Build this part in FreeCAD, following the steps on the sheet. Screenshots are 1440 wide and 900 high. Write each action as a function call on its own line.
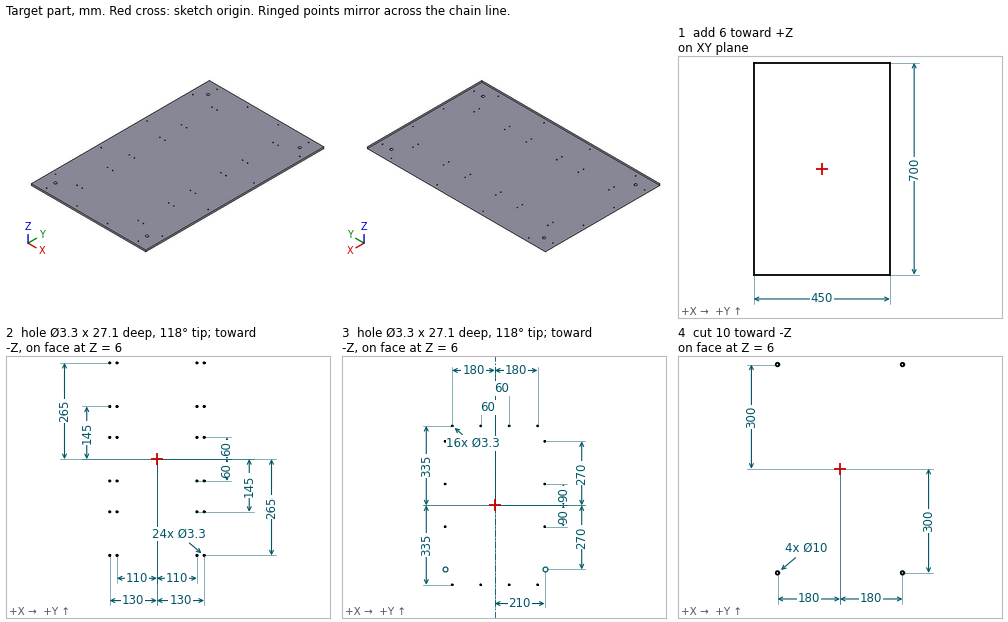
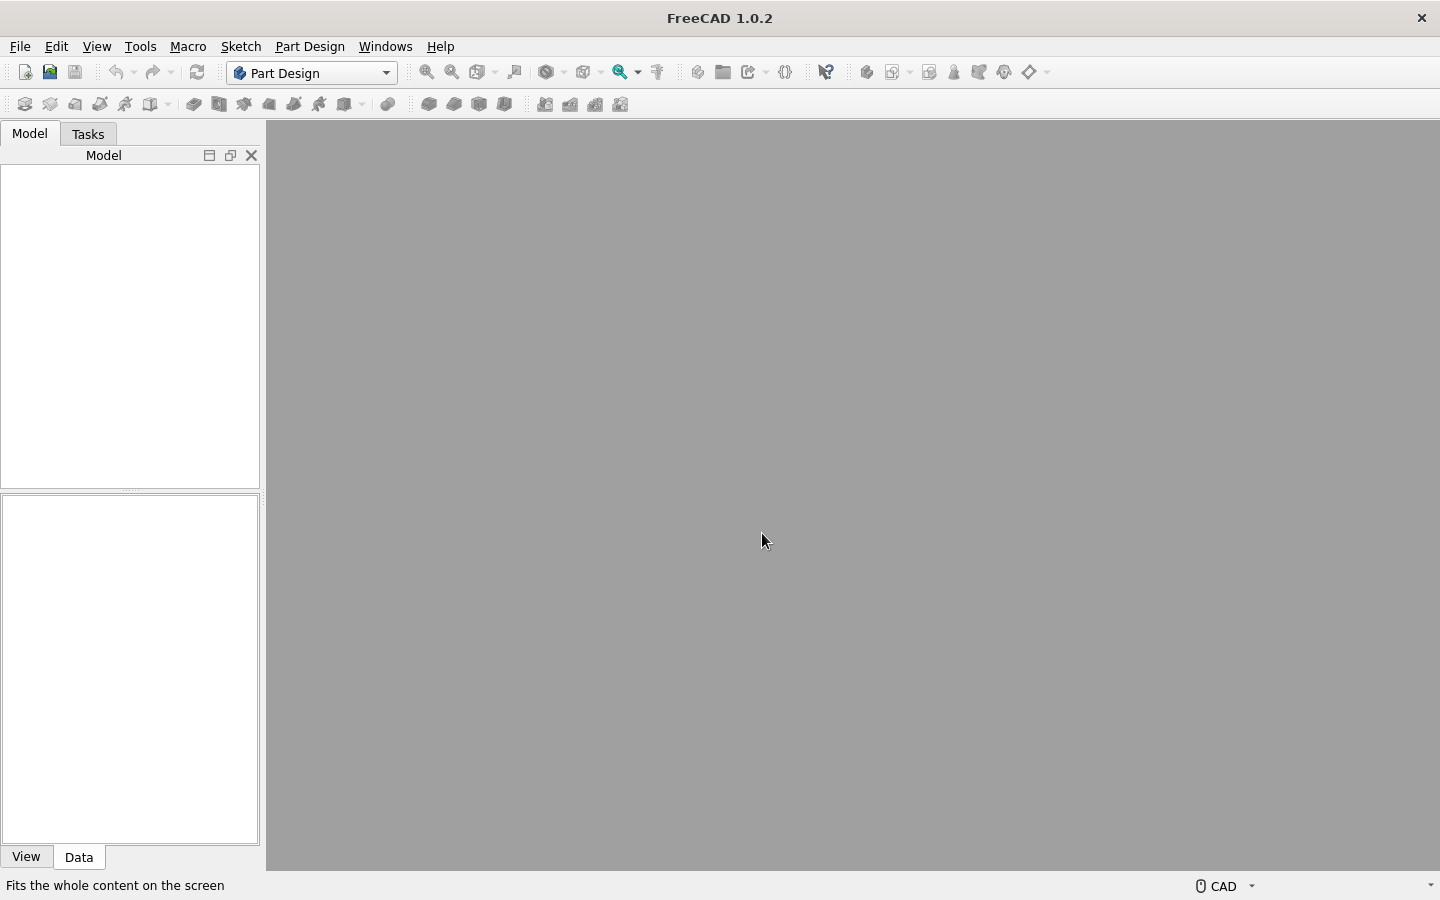
click(25, 72)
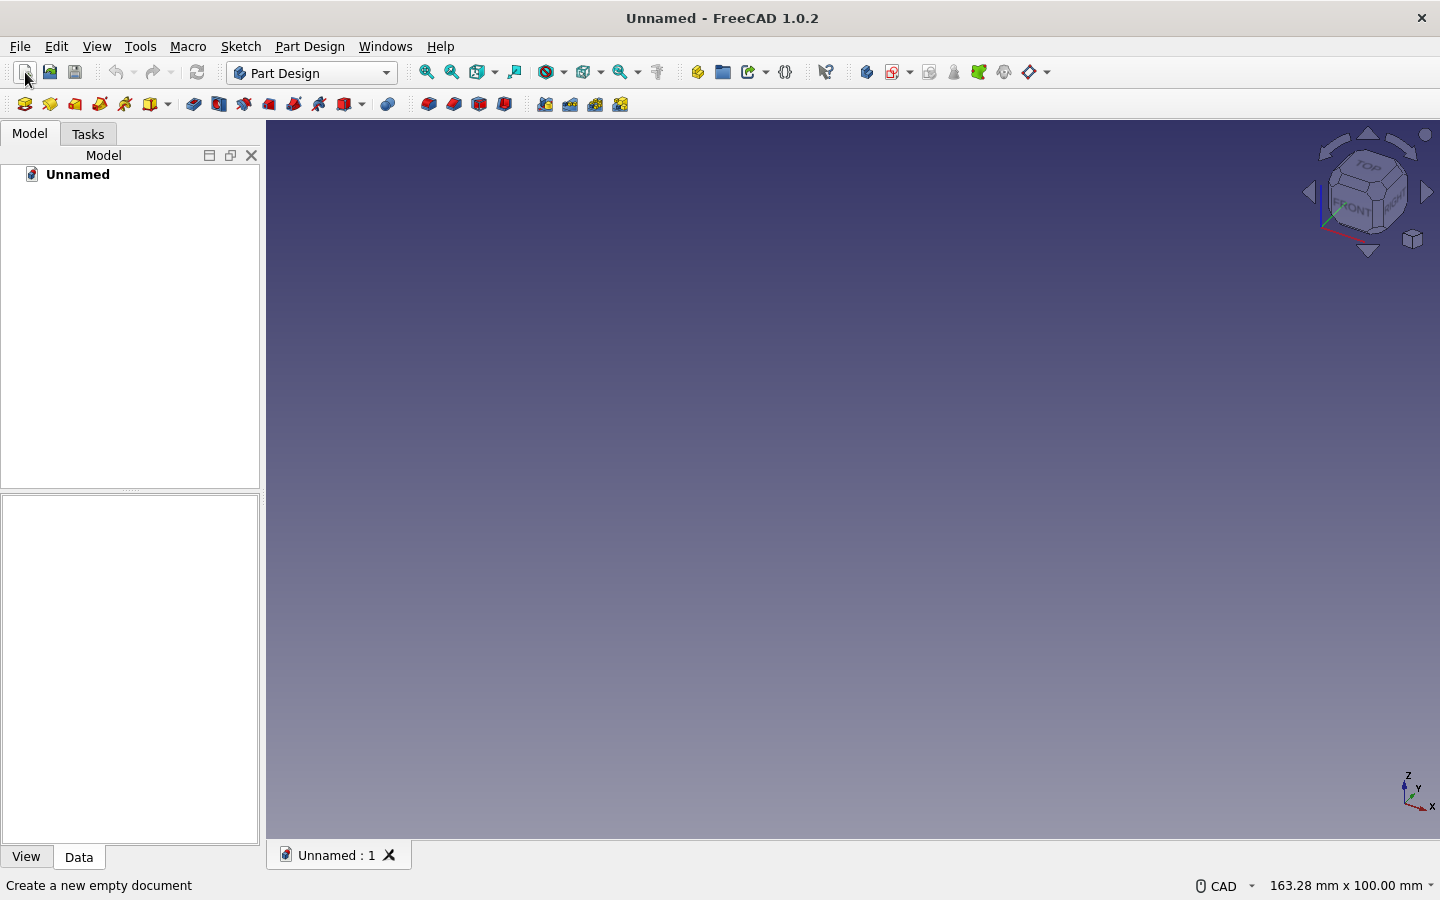
click(892, 72)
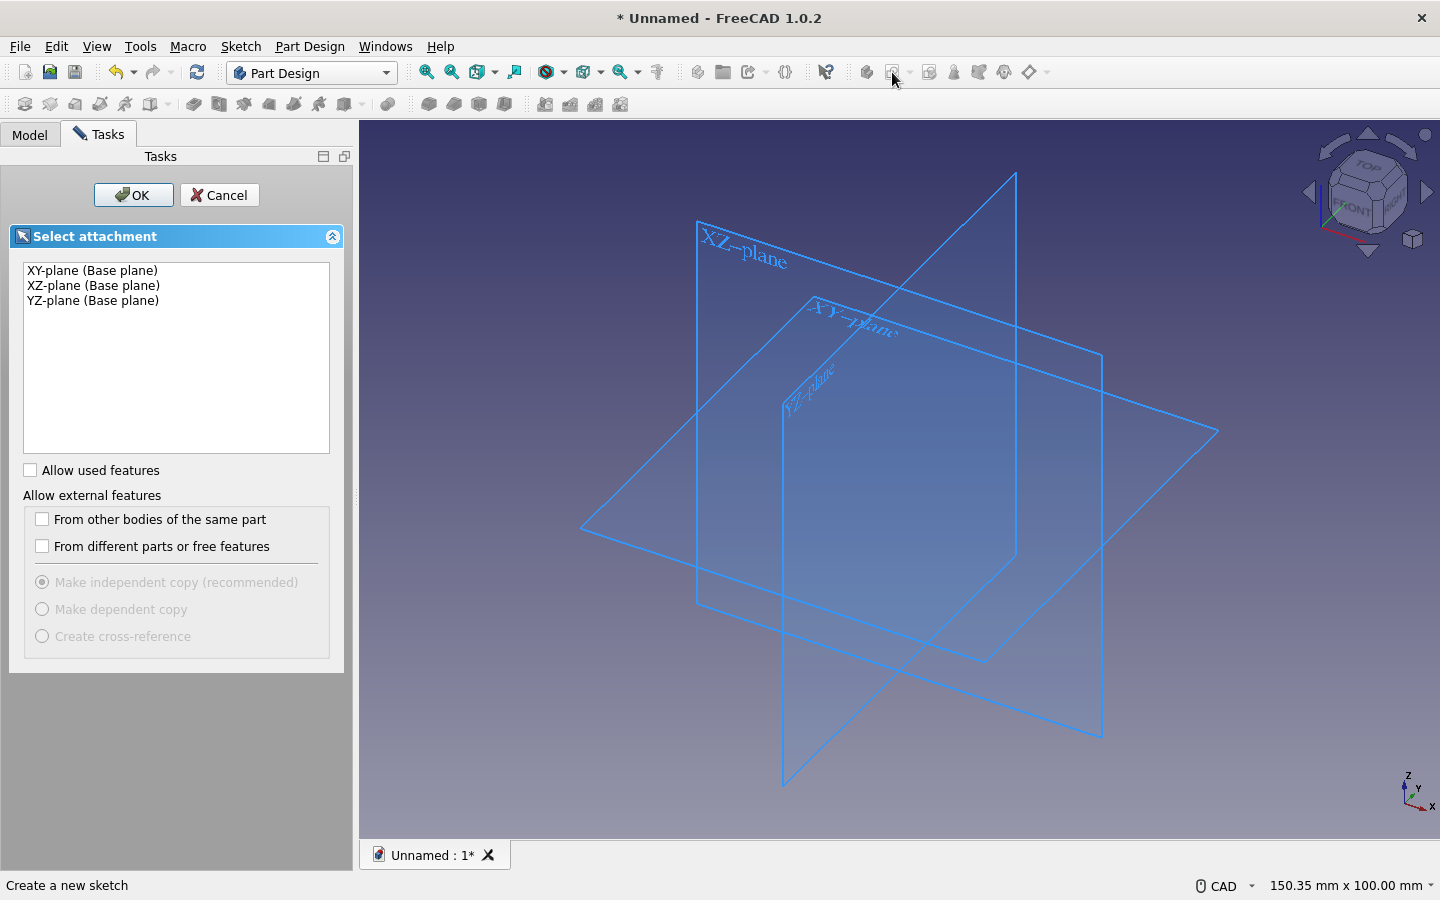
click(84, 270)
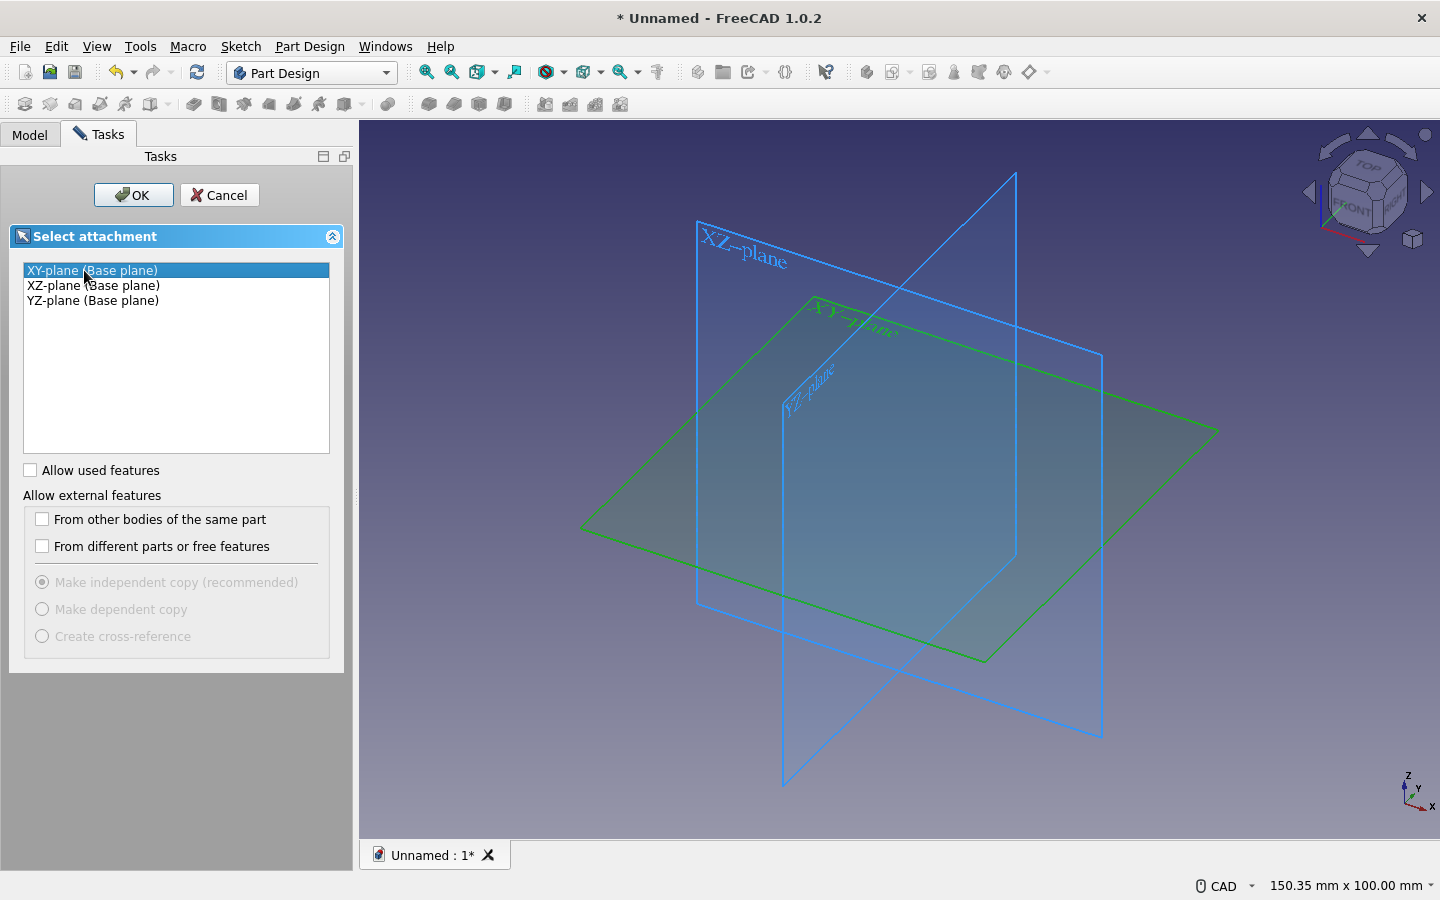
click(134, 195)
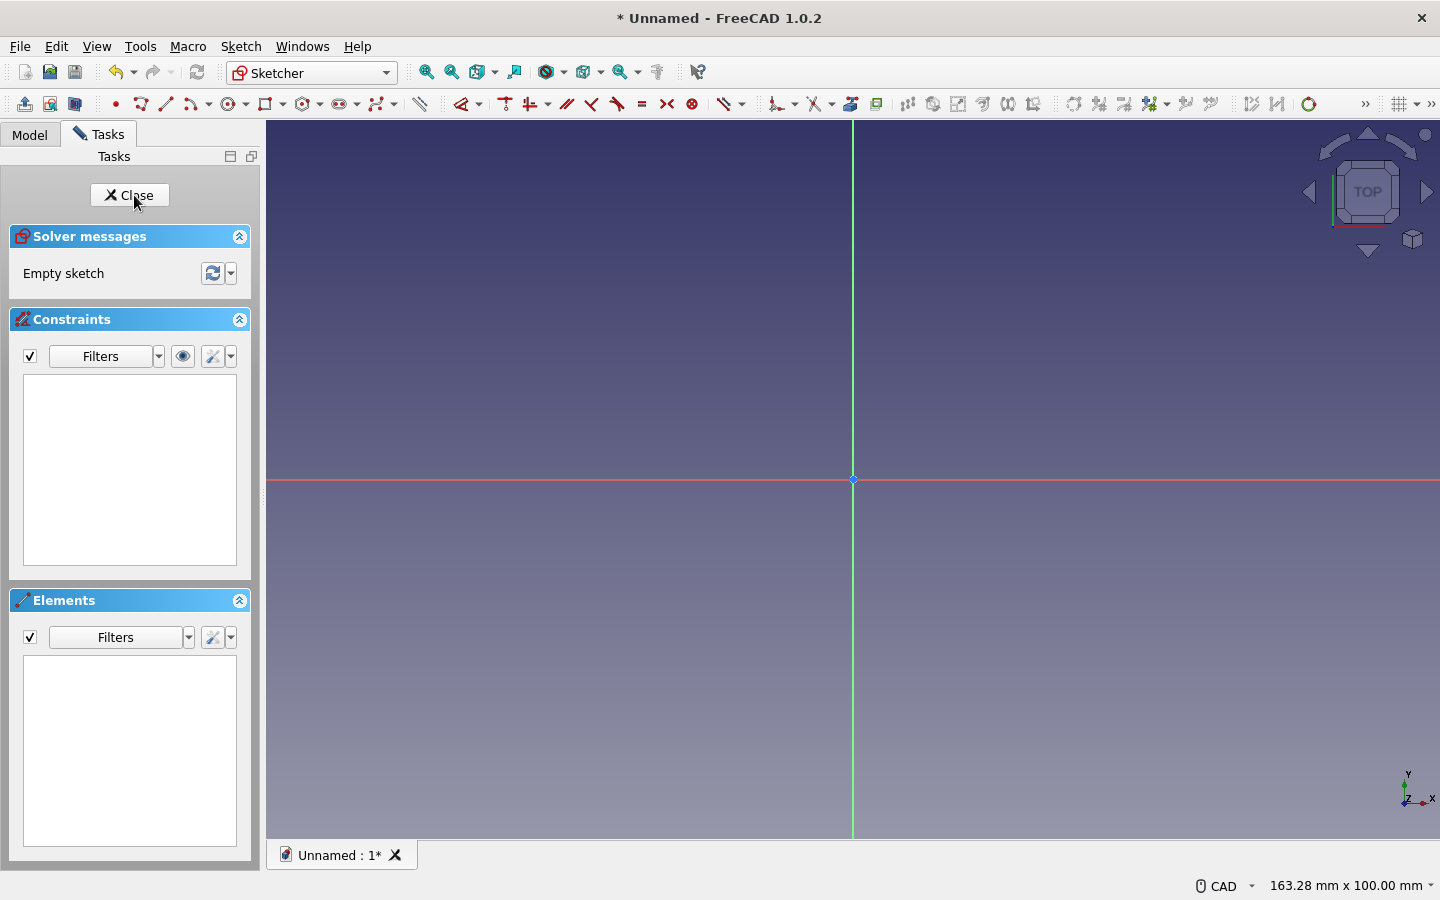
scroll(778, 479, down, 12)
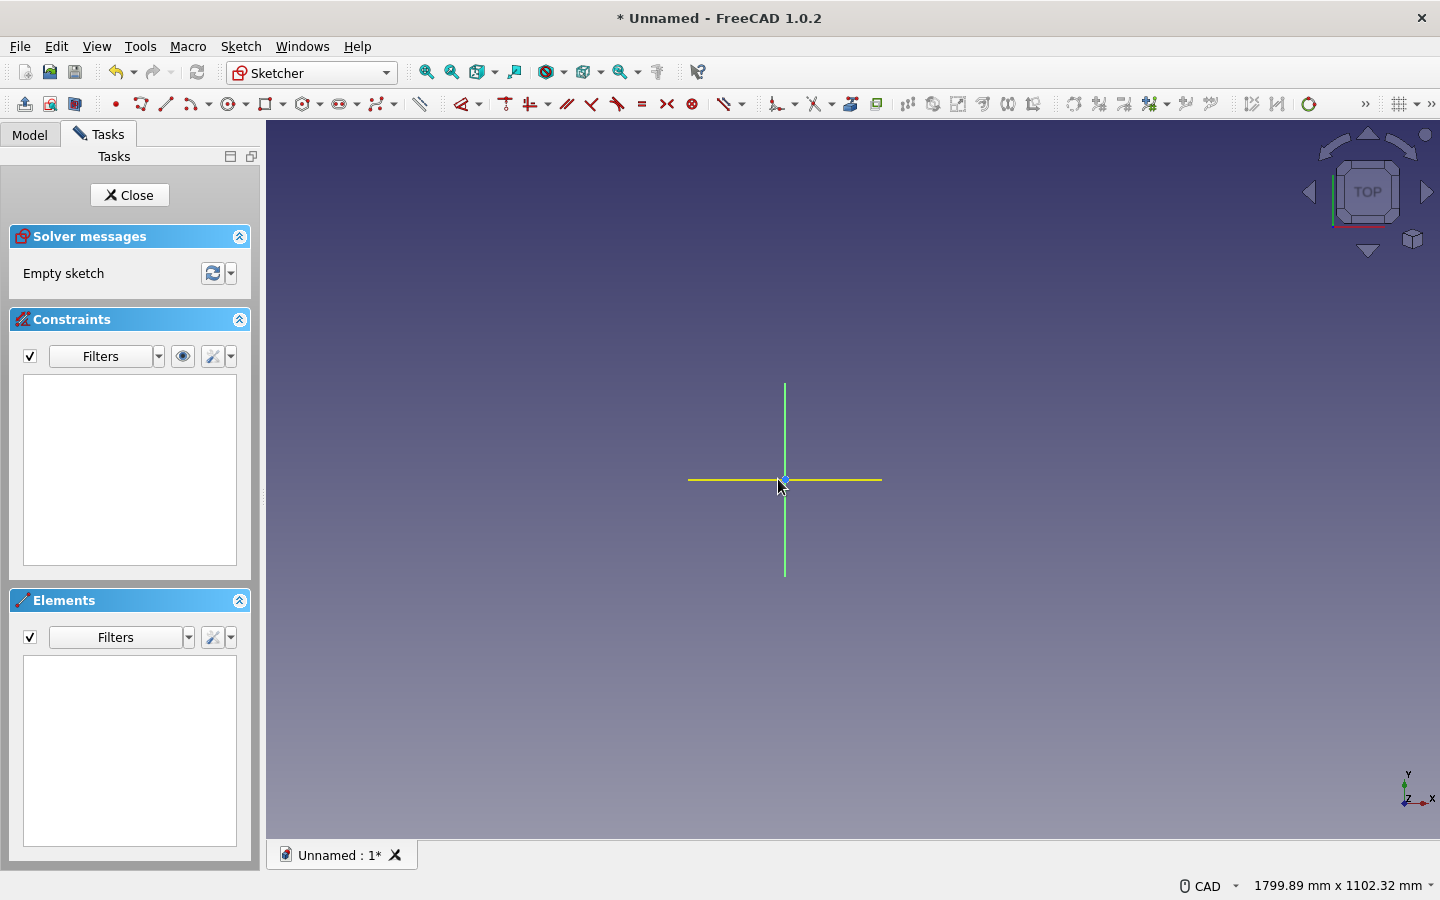
click(282, 104)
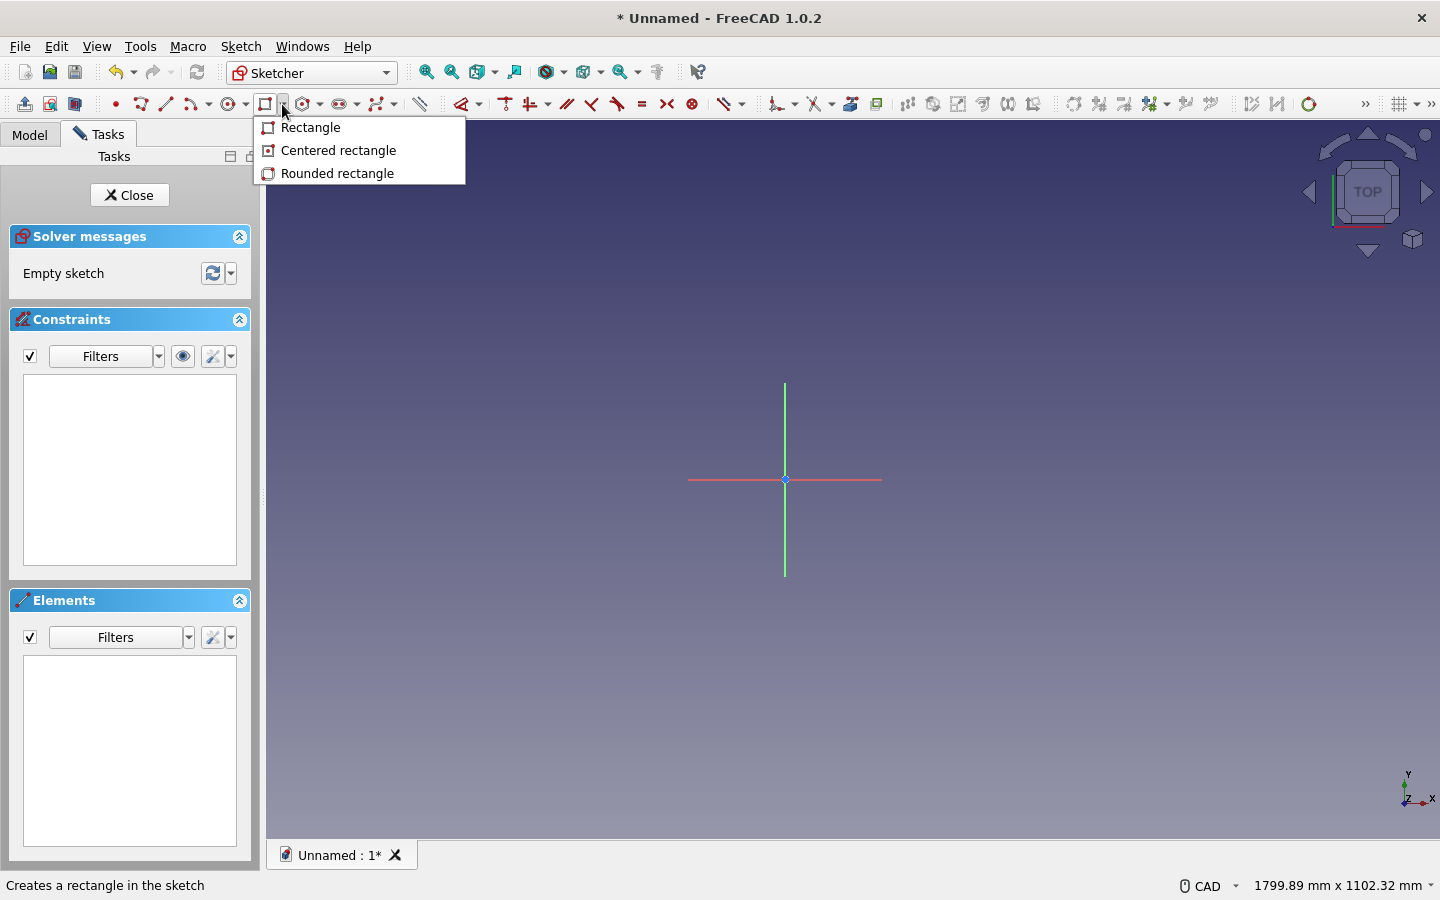
click(360, 150)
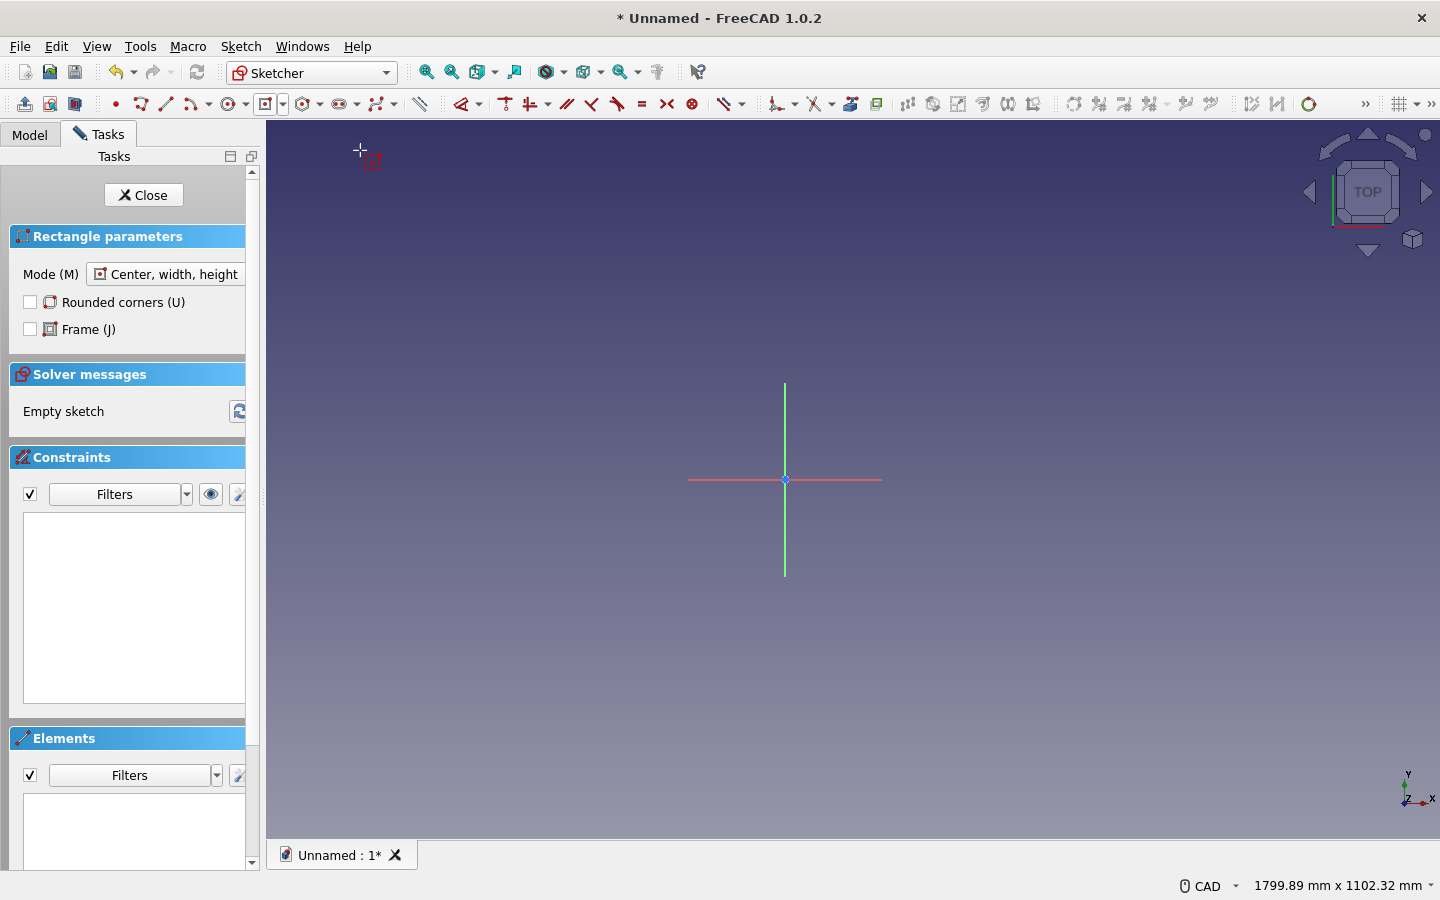
click(785, 480)
move(932, 251)